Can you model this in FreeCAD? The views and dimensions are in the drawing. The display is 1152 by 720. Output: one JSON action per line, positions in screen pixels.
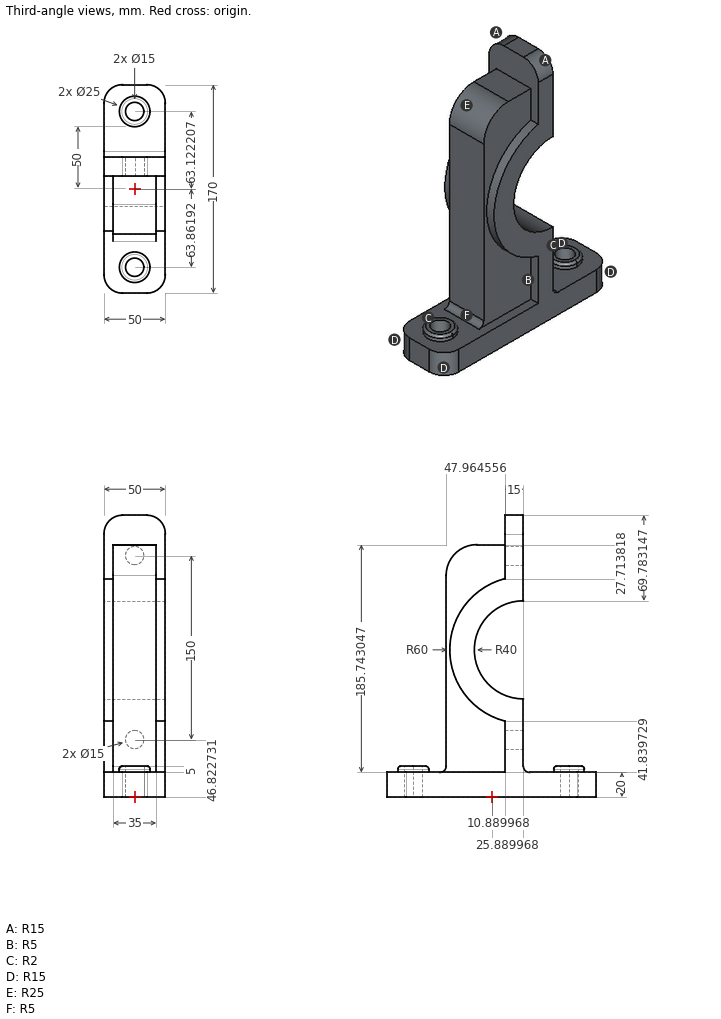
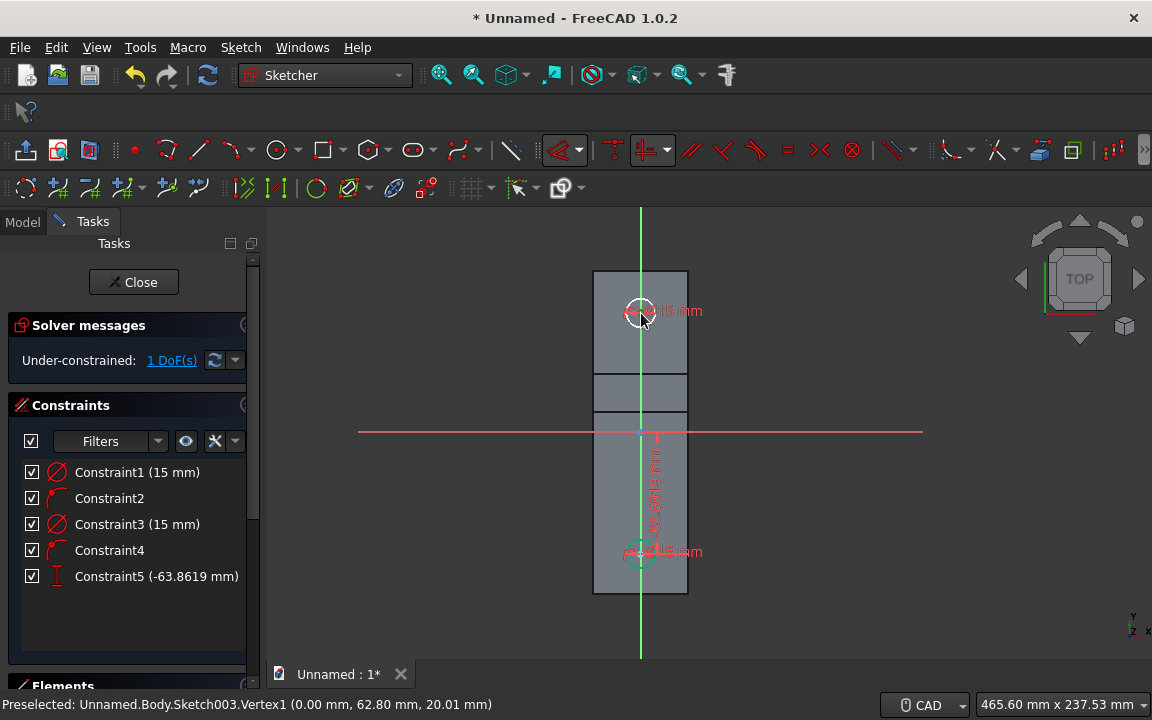
{"action": "left_click", "coordinate": [582, 150]}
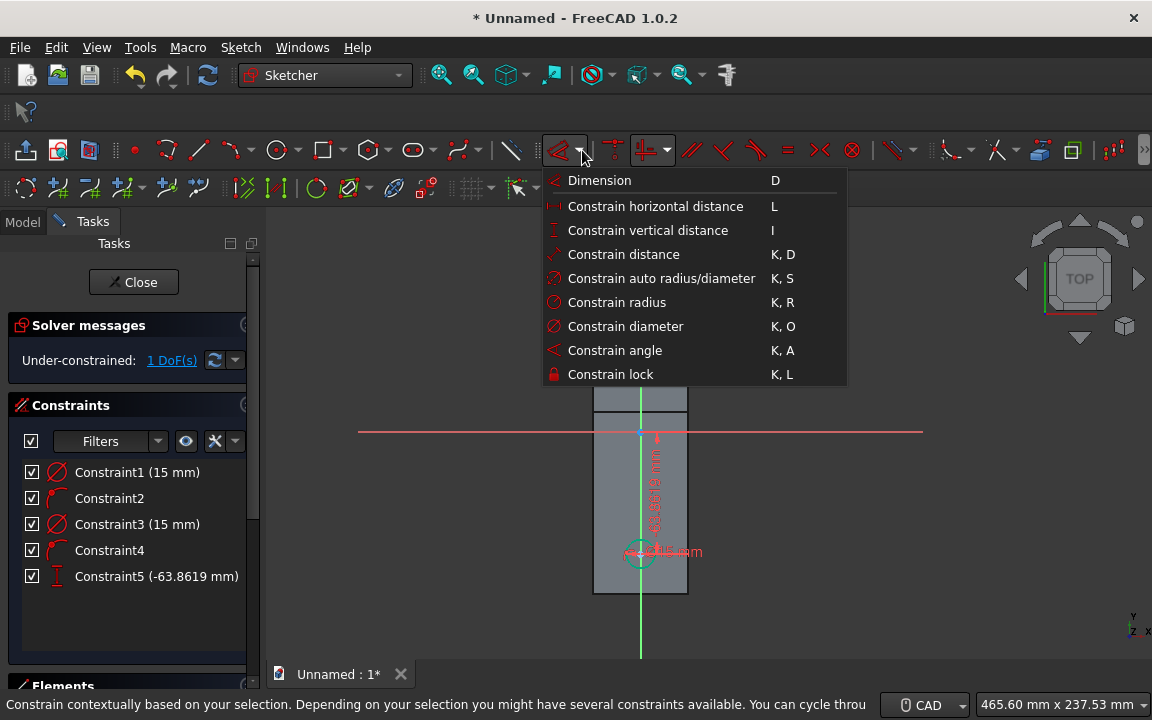
{"action": "left_click", "coordinate": [695, 230]}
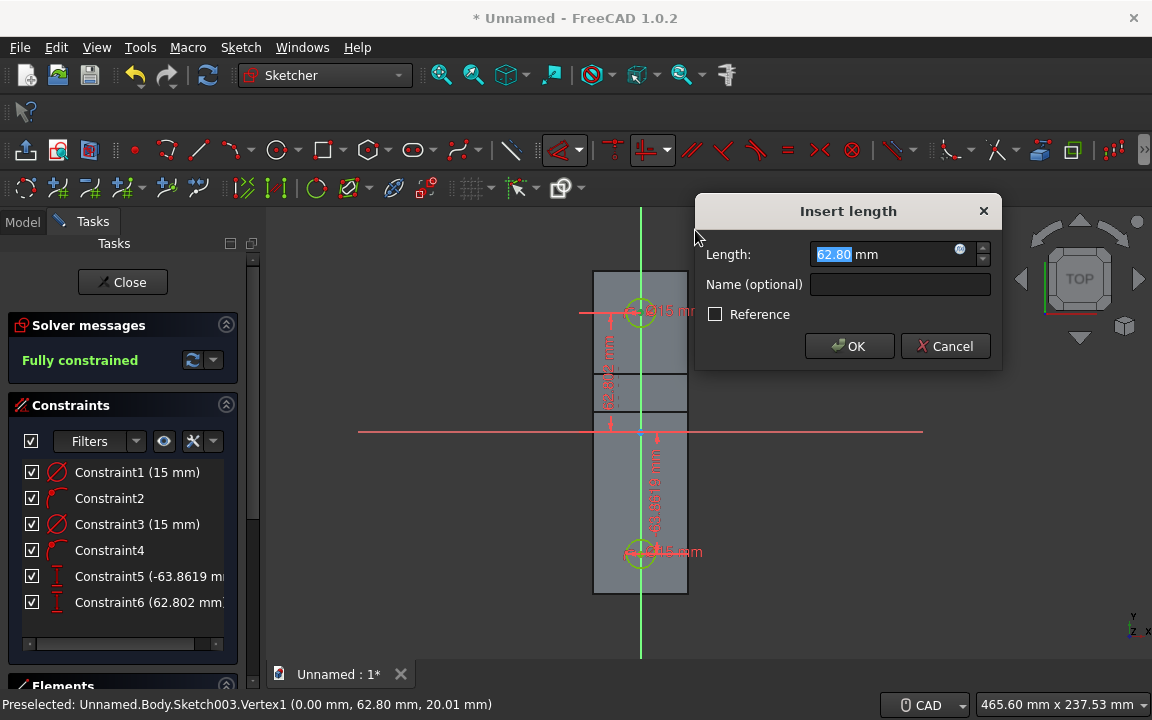
{"action": "type", "text": "63.122207"}
{"action": "key", "text": "Return"}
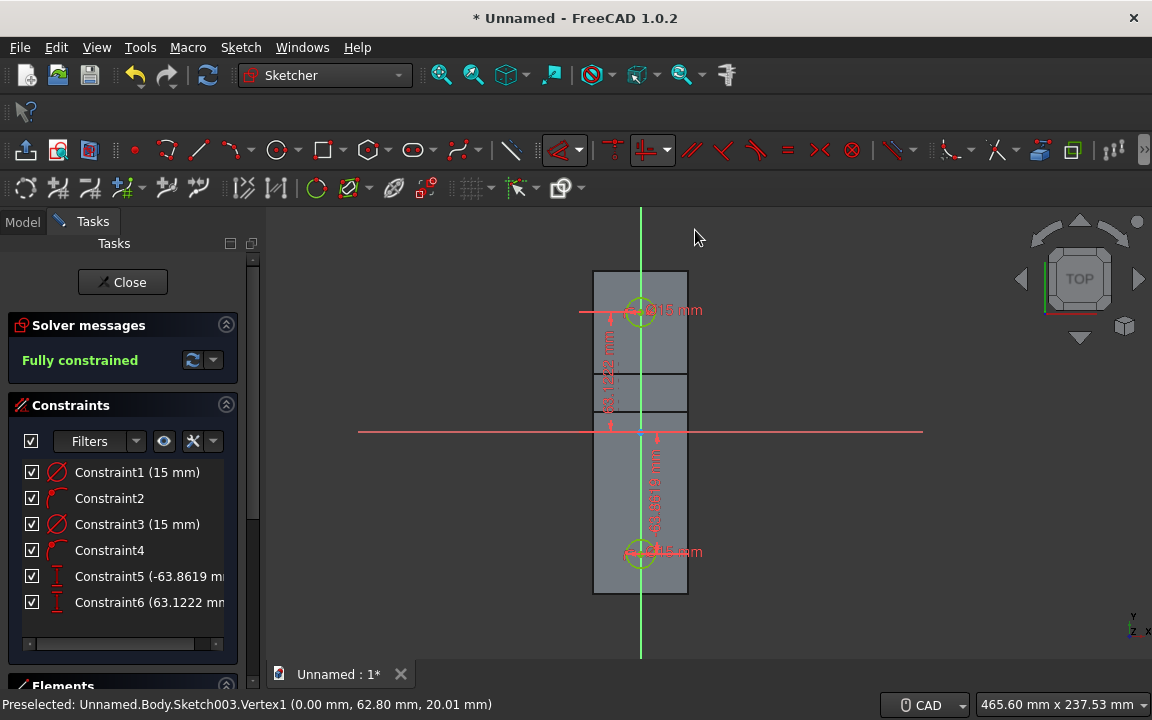
{"action": "left_click", "coordinate": [123, 282]}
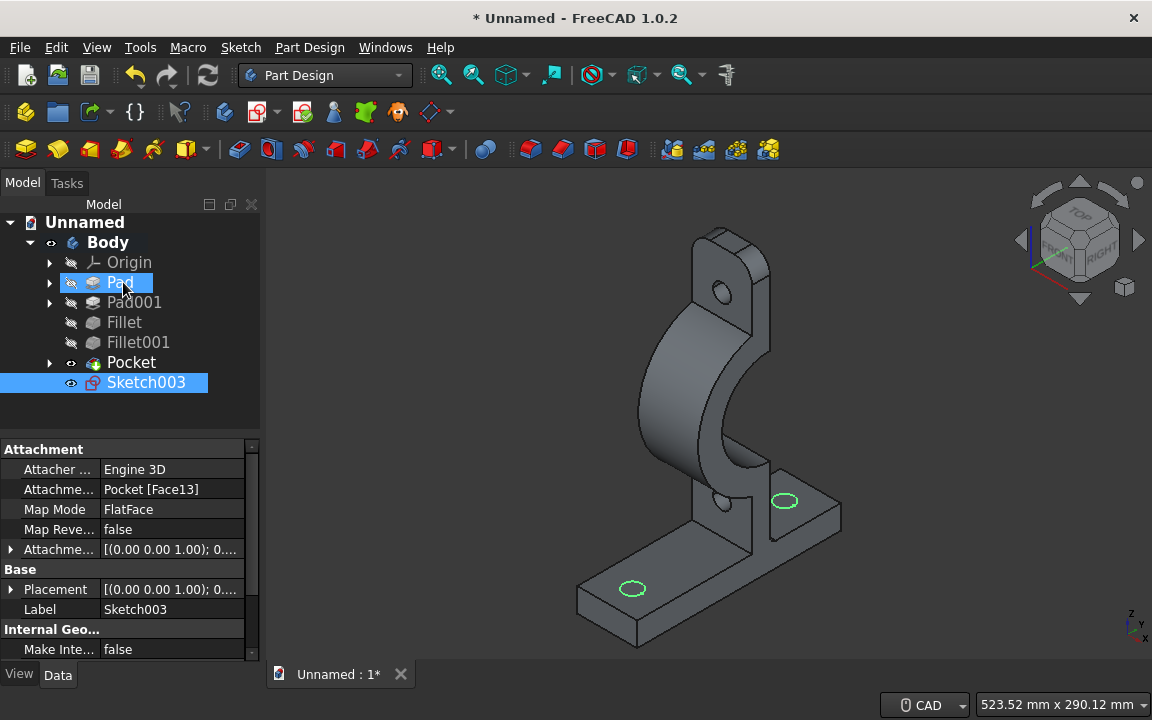
{"action": "left_click", "coordinate": [240, 150]}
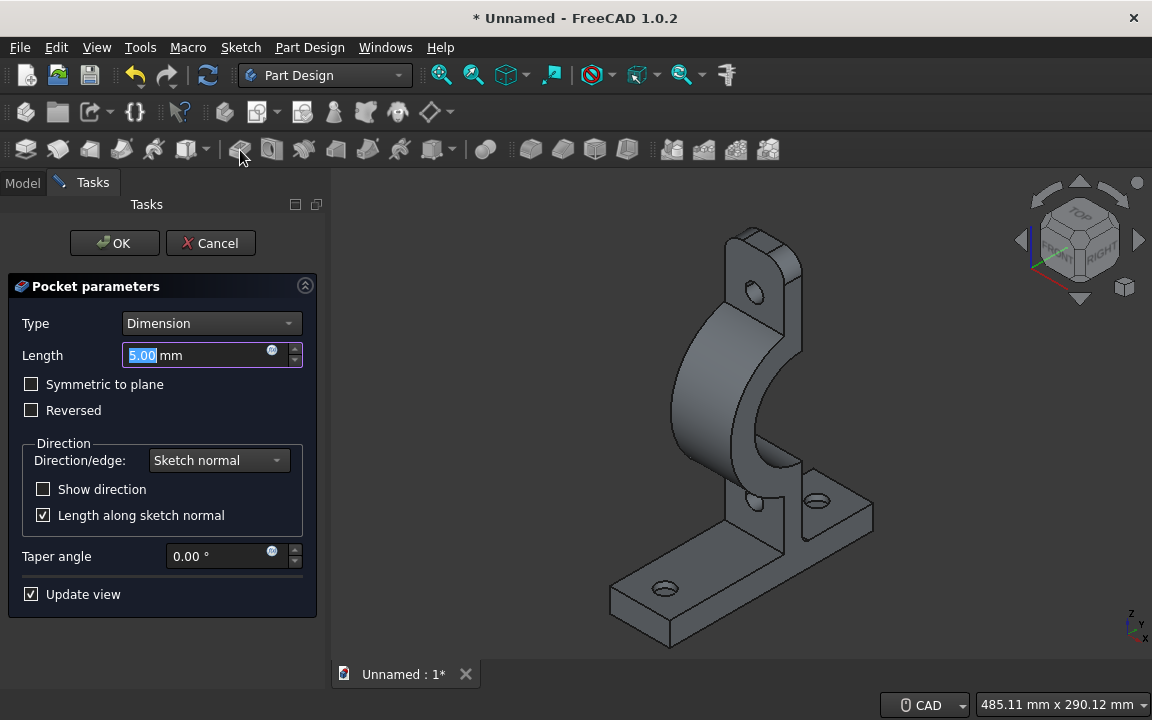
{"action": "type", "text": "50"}
{"action": "key", "text": "Tab"}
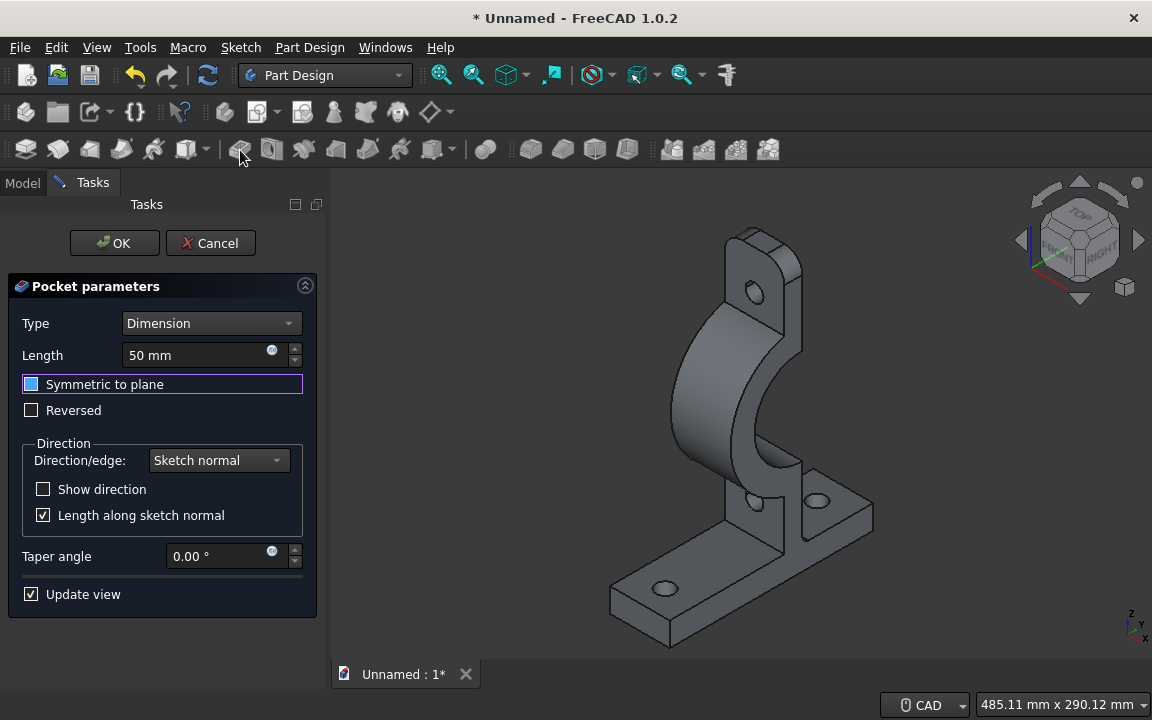
{"action": "left_click", "coordinate": [30, 384]}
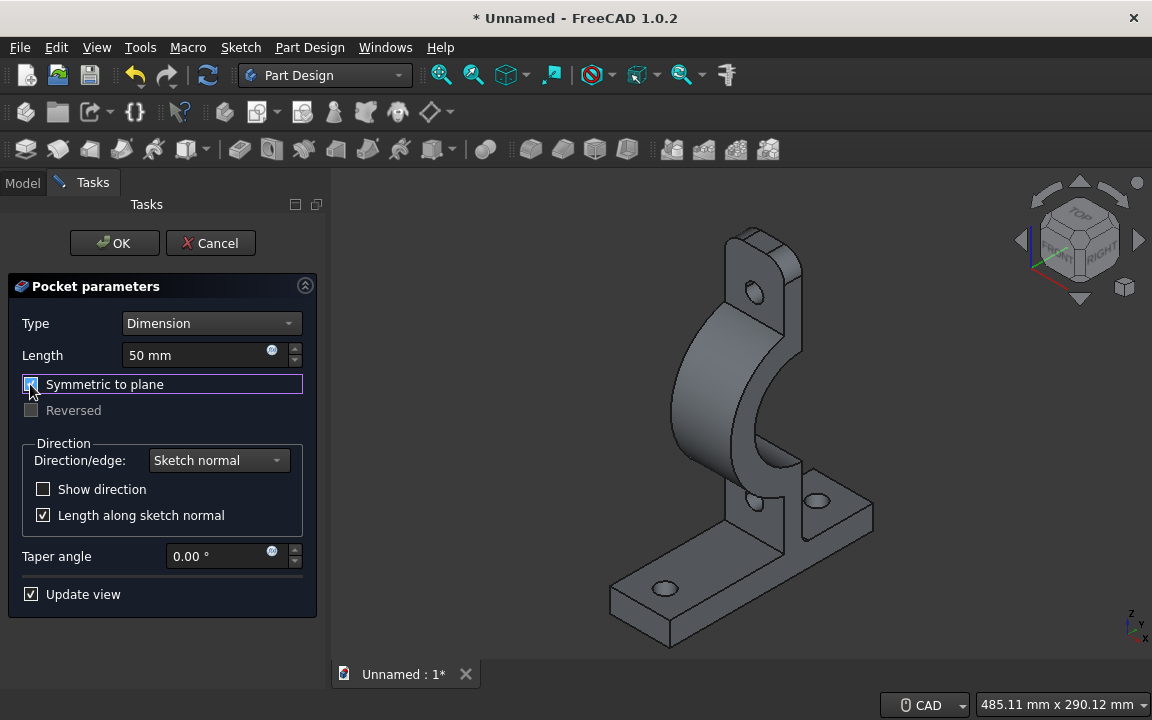
{"action": "left_click", "coordinate": [115, 243]}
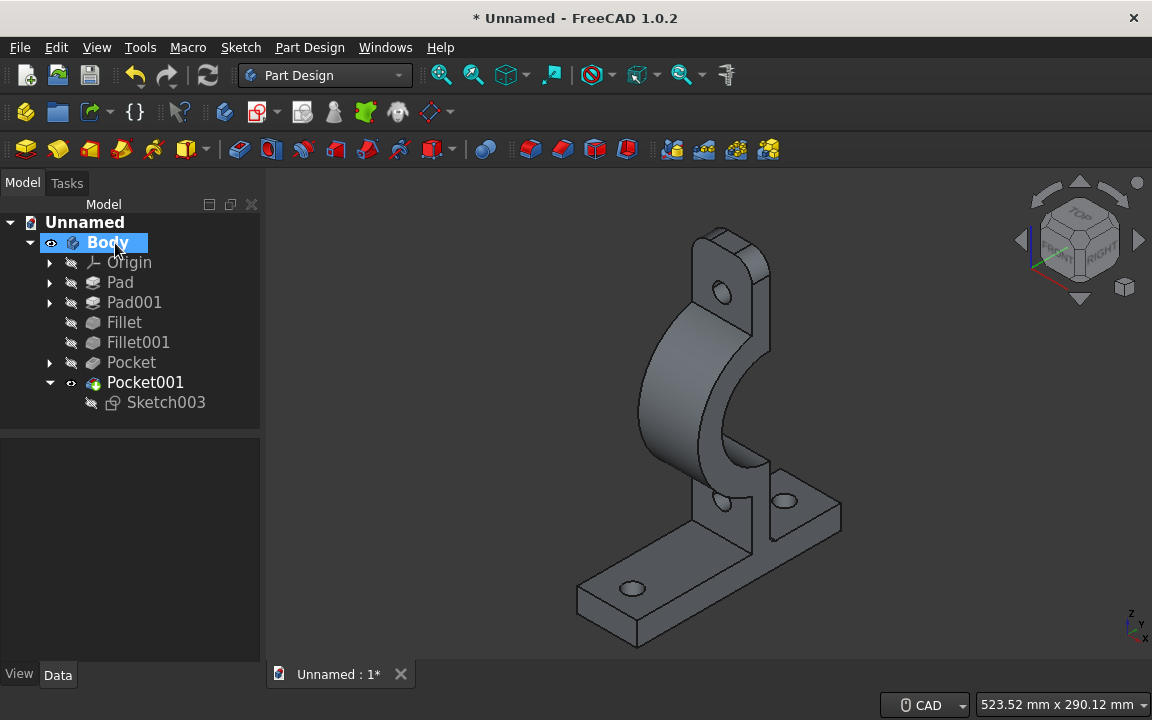
{"action": "left_click", "coordinate": [50, 263]}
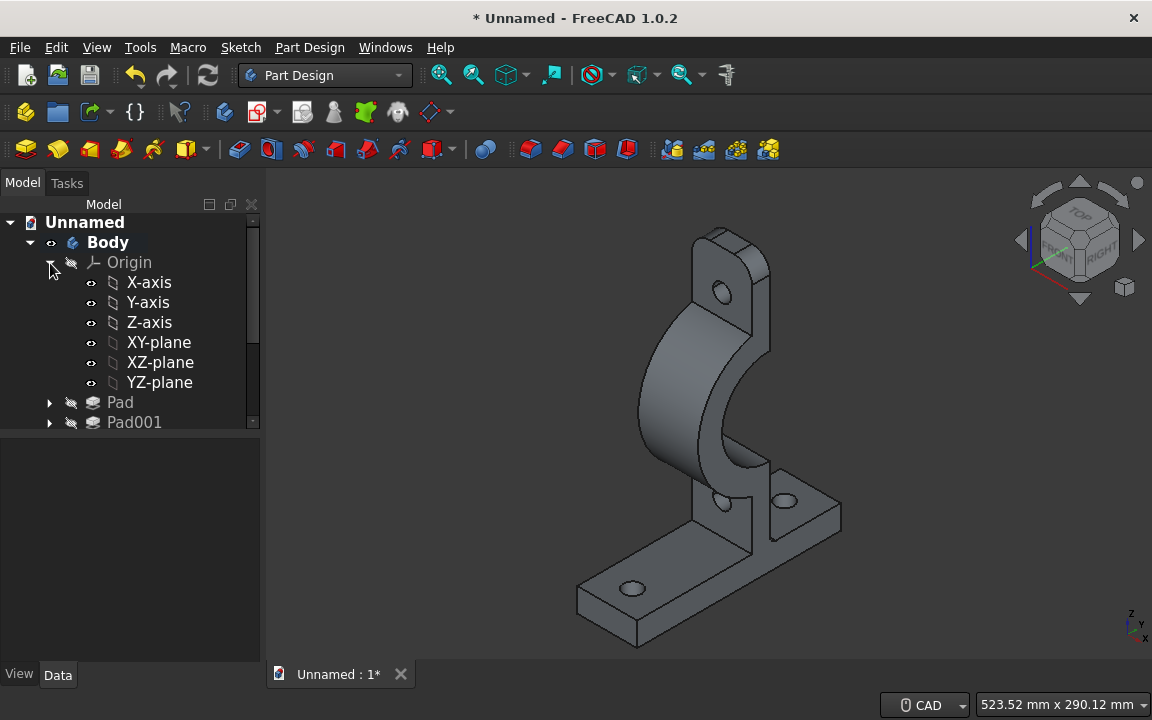
{"action": "left_click", "coordinate": [136, 343]}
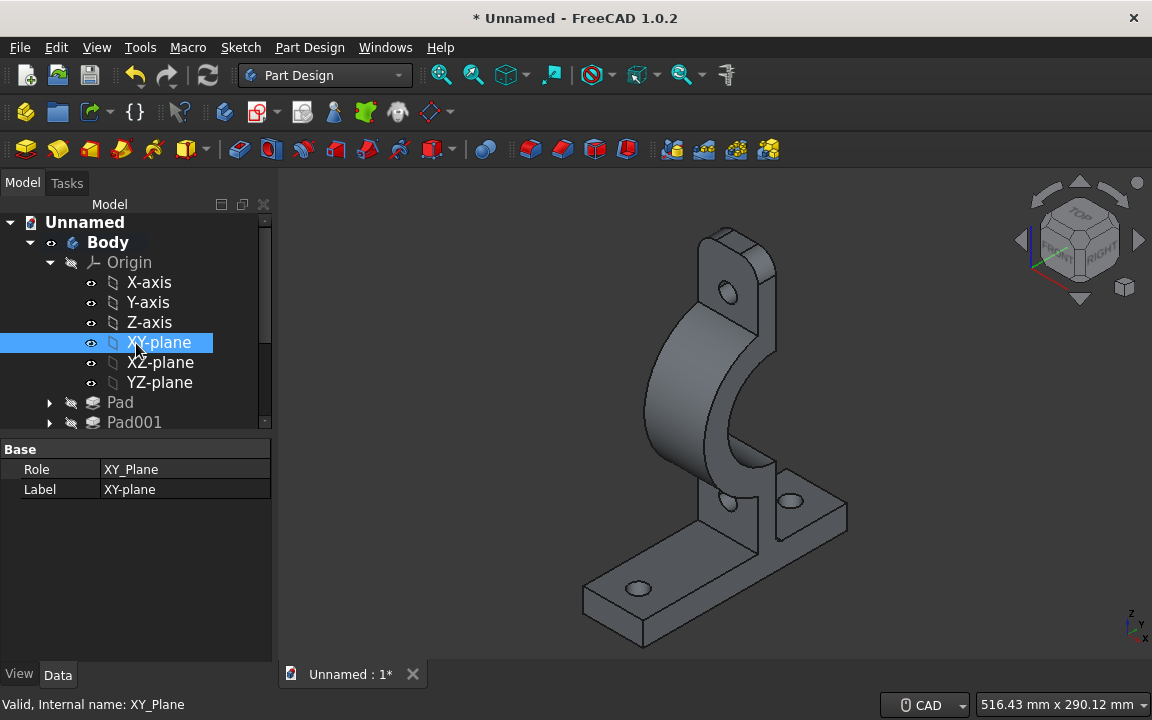
{"action": "left_click", "coordinate": [430, 112]}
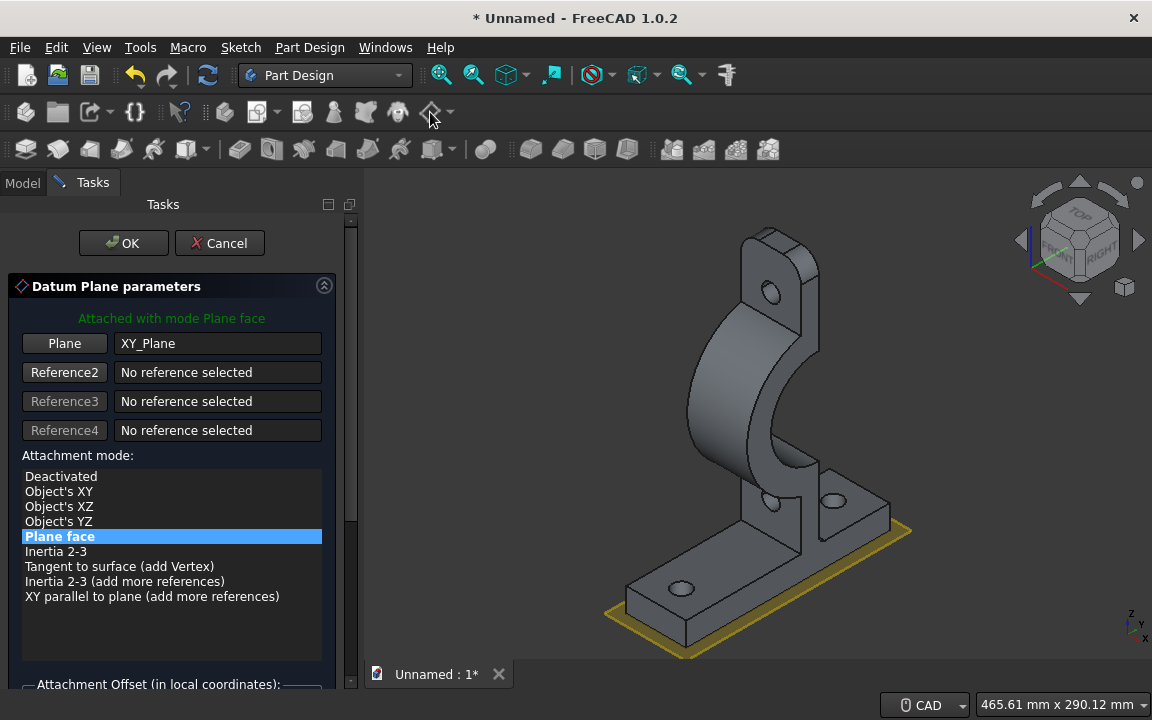
{"action": "scroll", "coordinate": [351, 451], "scroll_direction": "down", "scroll_amount": 3}